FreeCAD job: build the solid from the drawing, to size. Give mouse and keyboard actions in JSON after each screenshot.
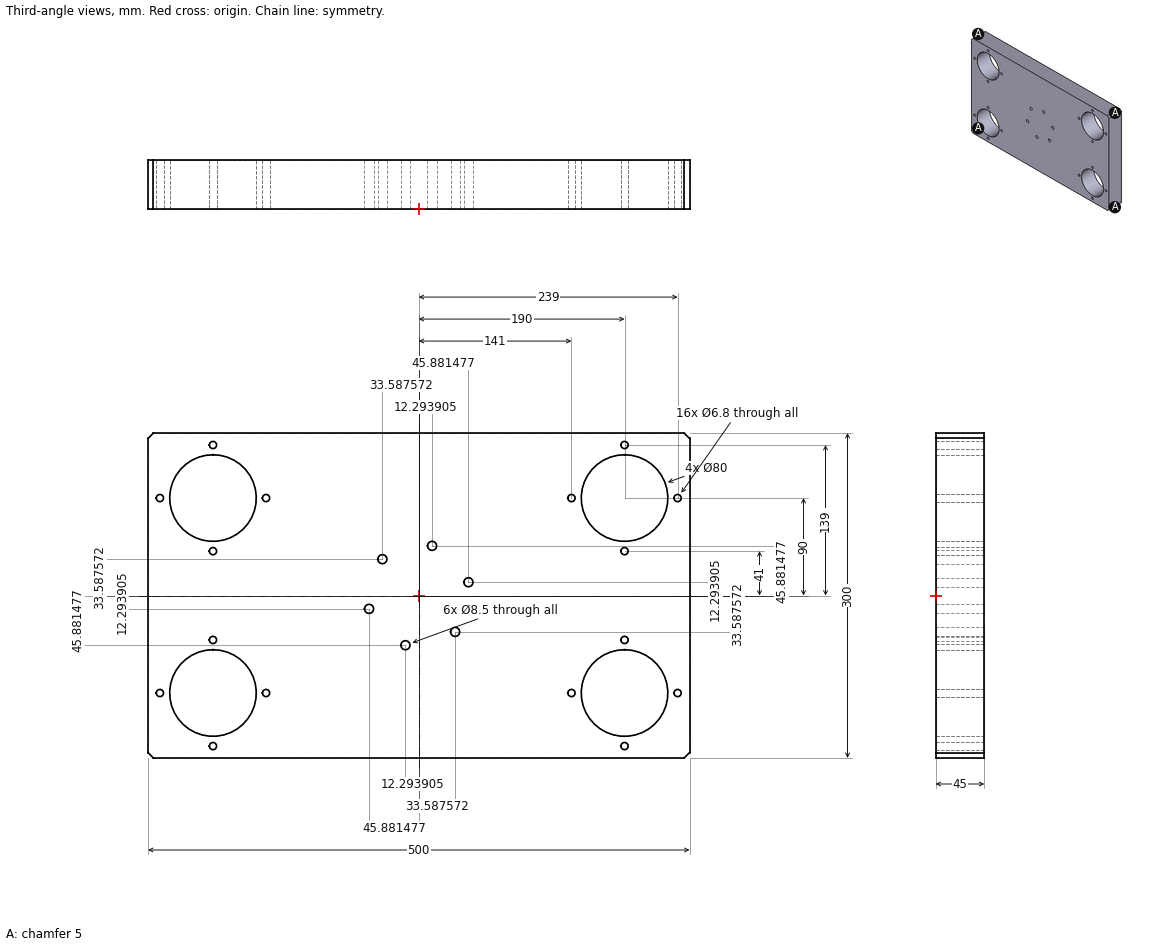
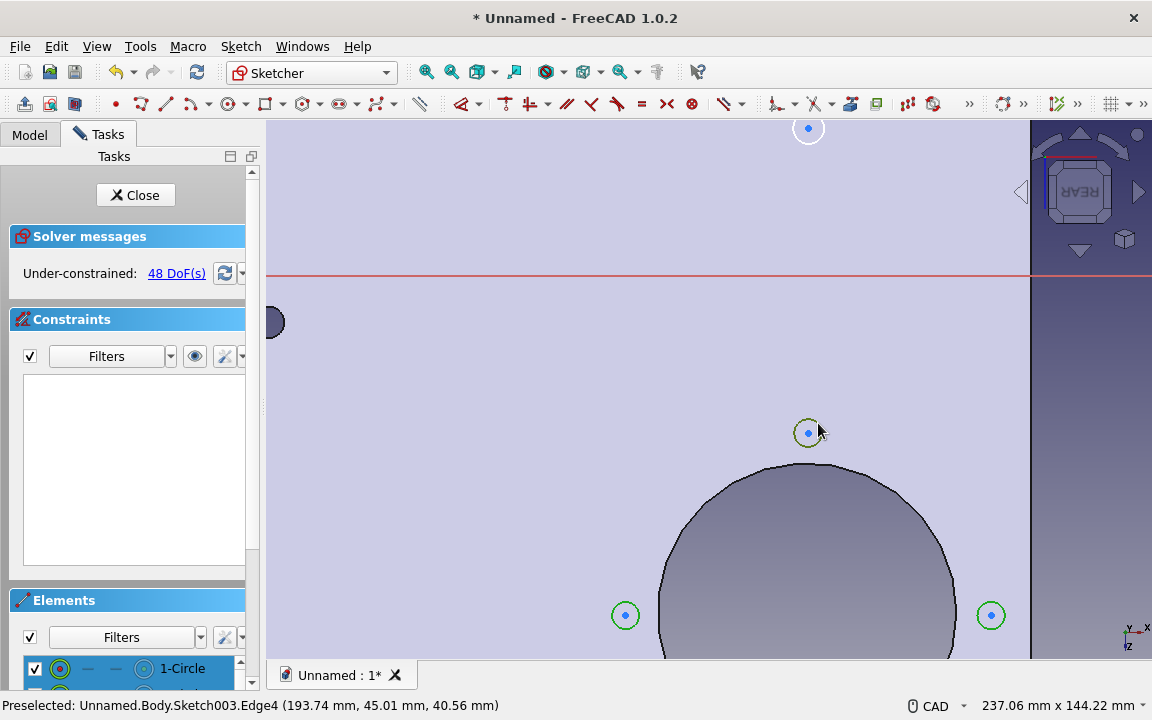
{"action": "scroll", "coordinate": [818, 427], "scroll_direction": "down", "scroll_amount": 7}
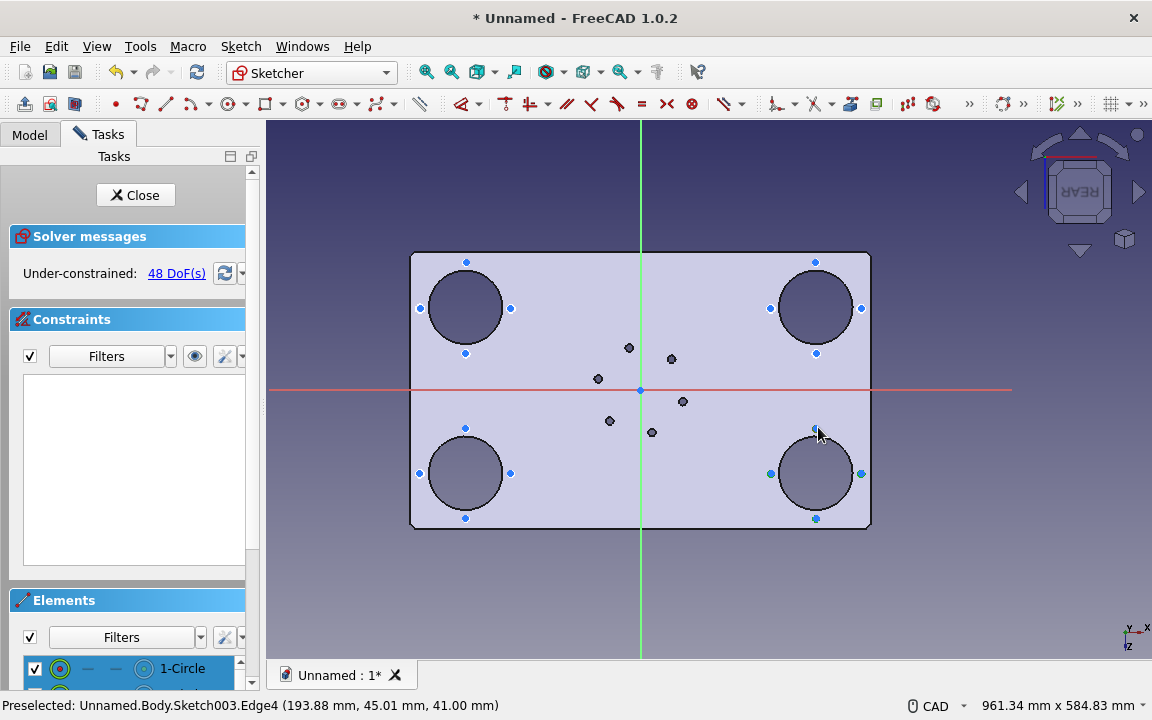
{"action": "scroll", "coordinate": [864, 306], "scroll_direction": "up", "scroll_amount": 7}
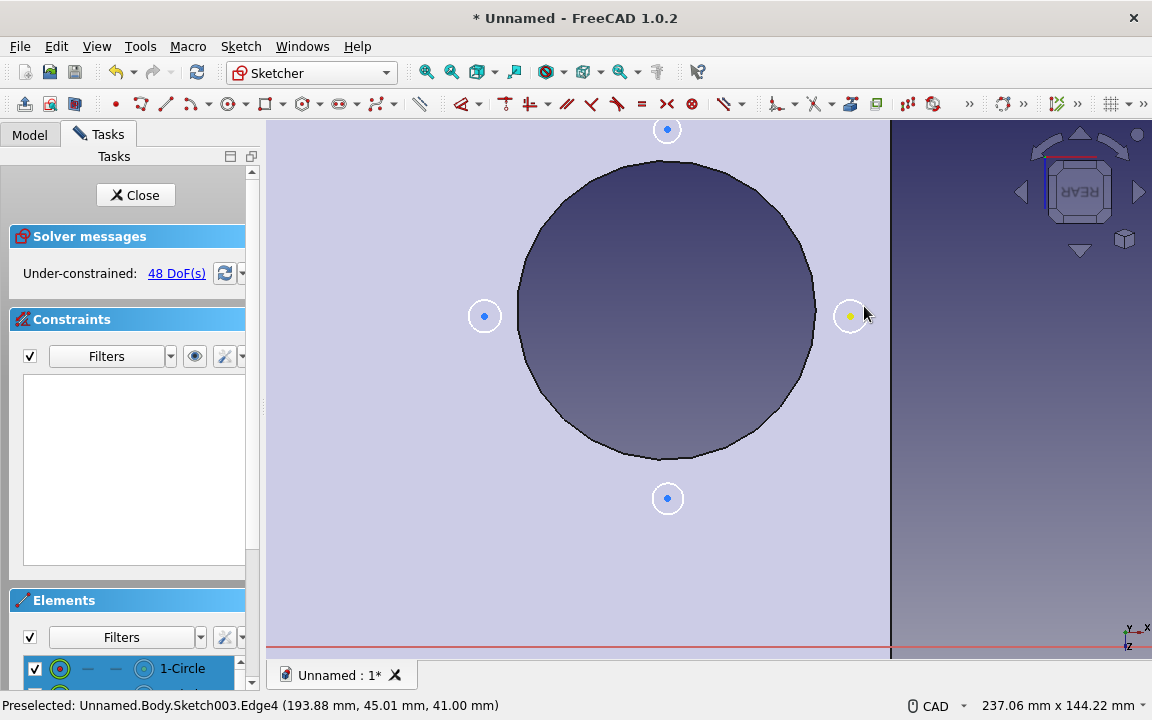
{"action": "left_click", "coordinate": [862, 305]}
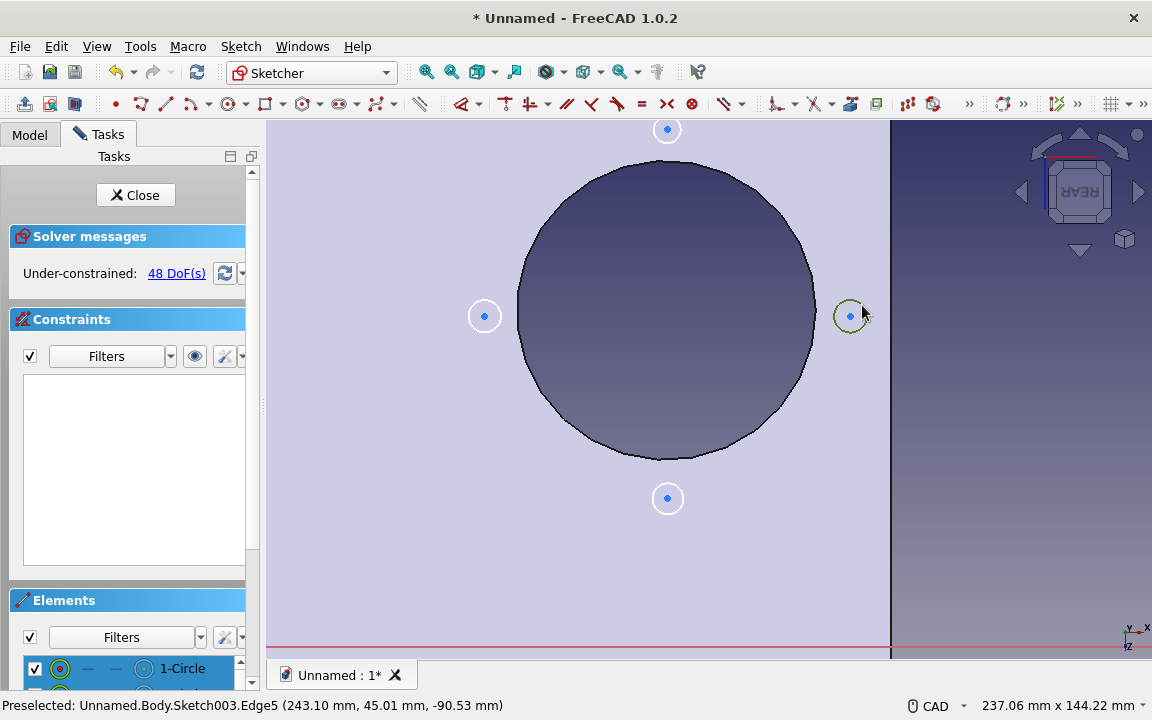
{"action": "left_click", "coordinate": [679, 488]}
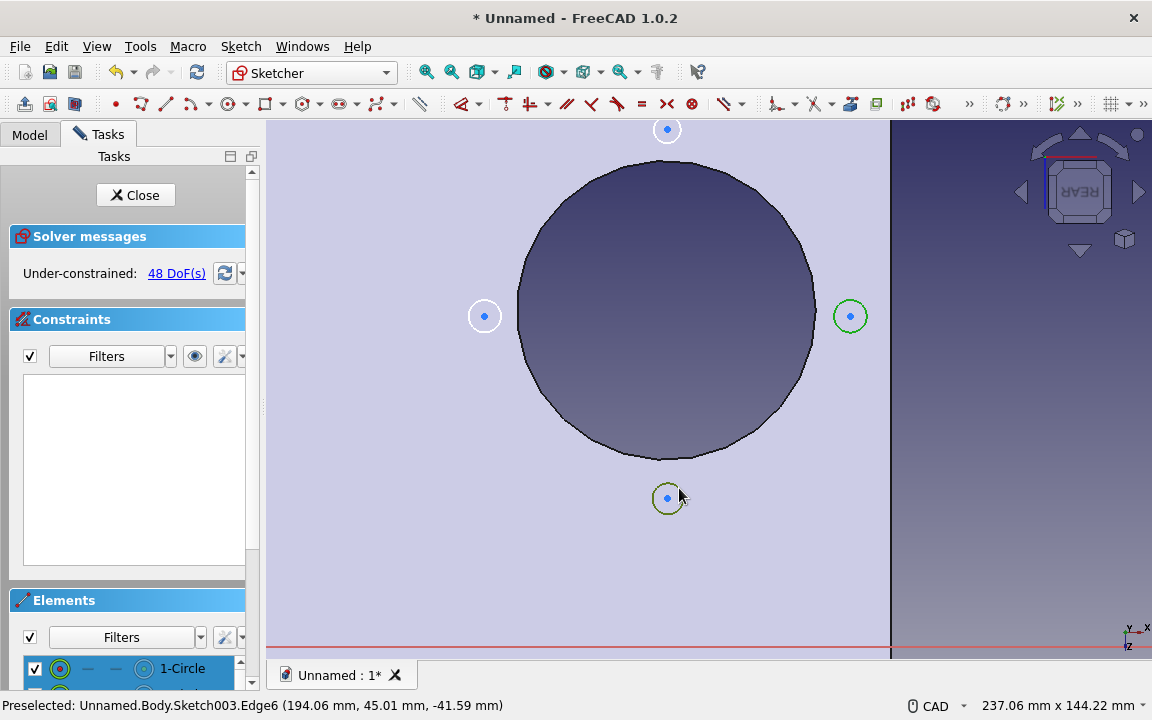
{"action": "left_click", "coordinate": [496, 305]}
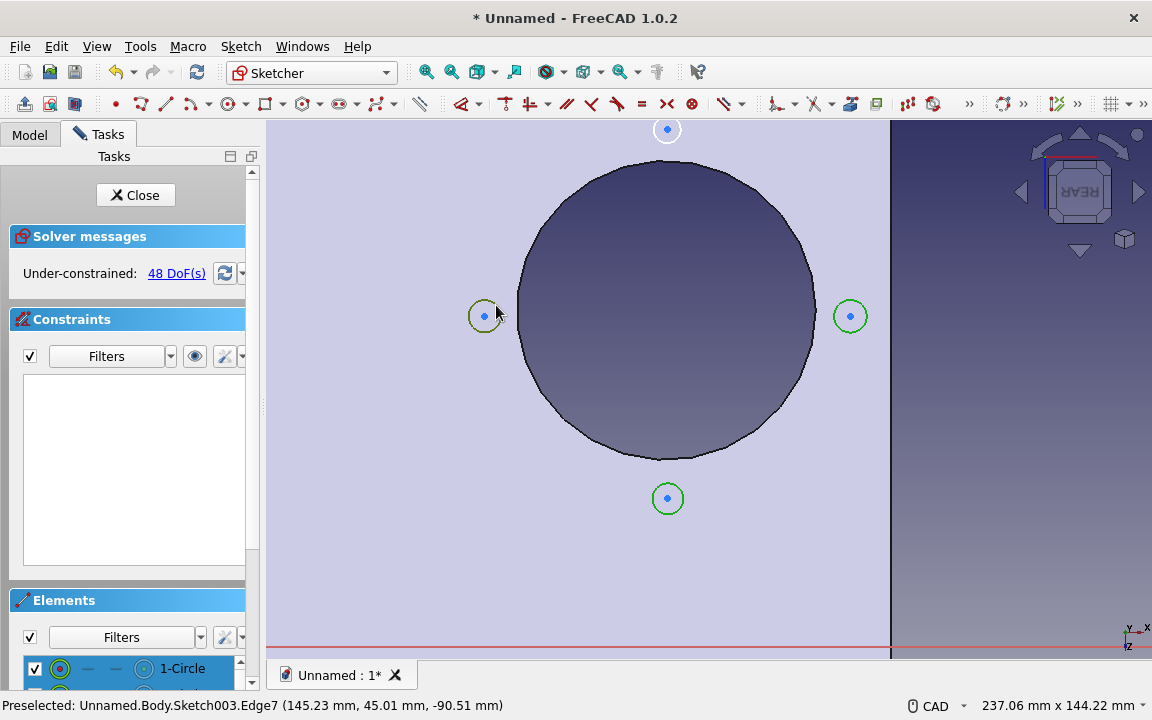
{"action": "scroll", "coordinate": [864, 305], "scroll_direction": "down", "scroll_amount": 7}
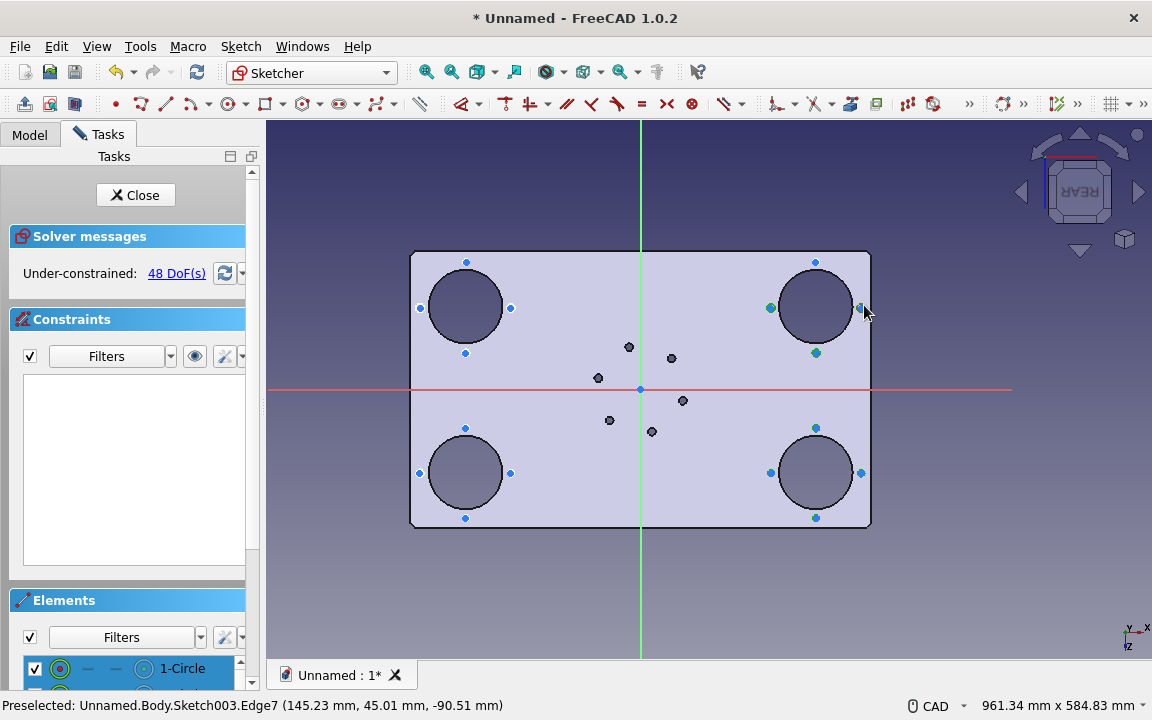
{"action": "scroll", "coordinate": [818, 260], "scroll_direction": "up", "scroll_amount": 8}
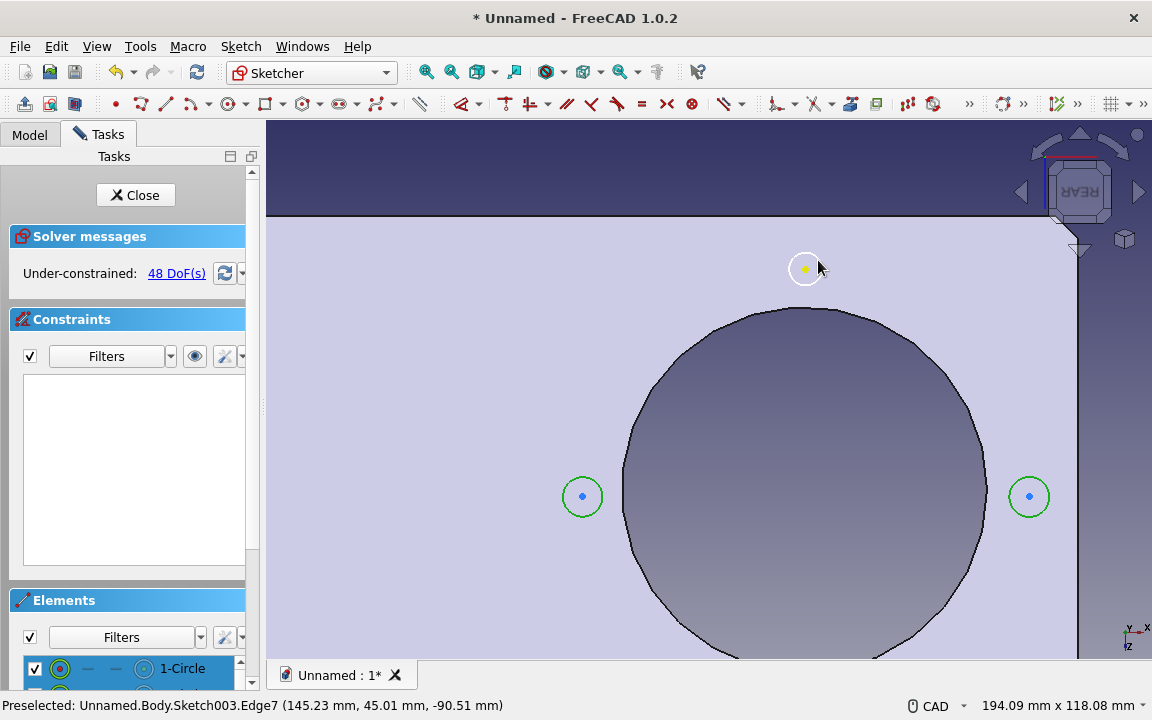
{"action": "left_click", "coordinate": [817, 257]}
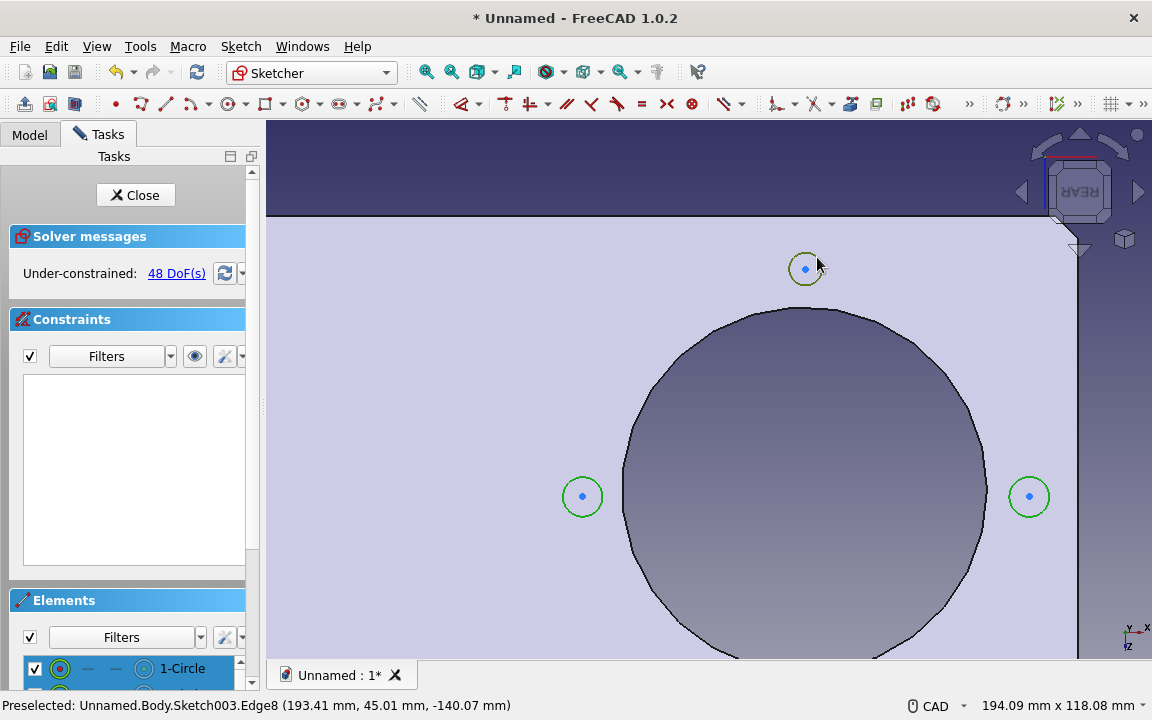
{"action": "scroll", "coordinate": [818, 260], "scroll_direction": "down", "scroll_amount": 8}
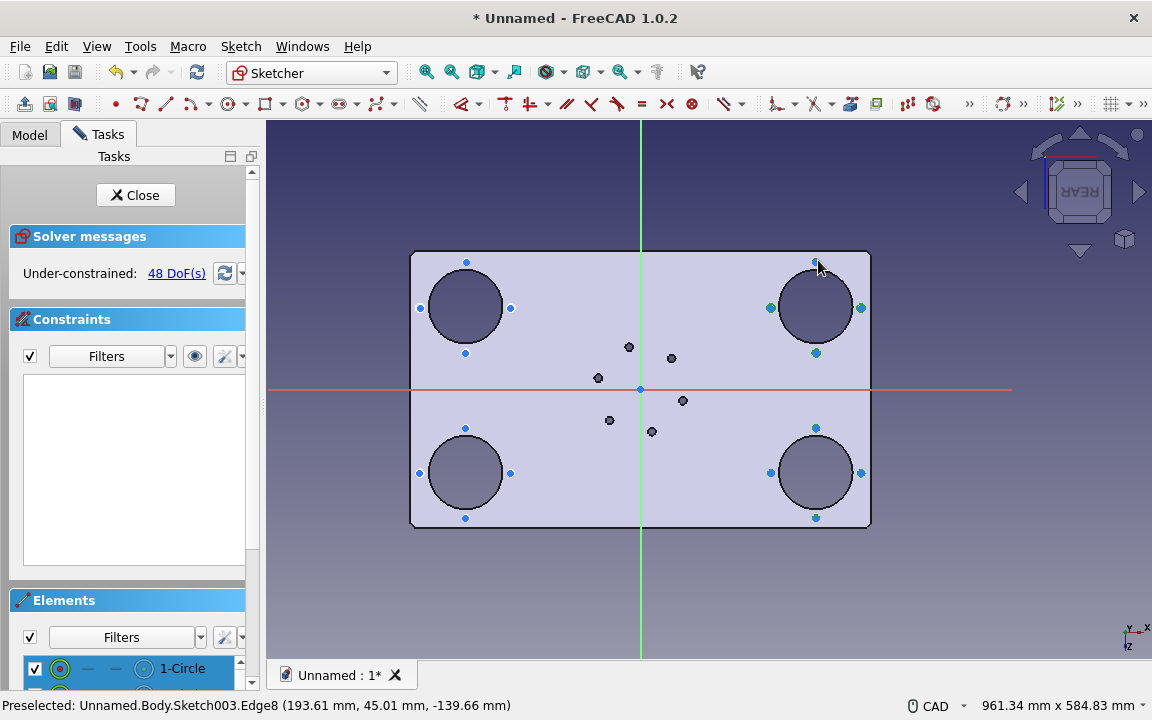
{"action": "scroll", "coordinate": [513, 471], "scroll_direction": "up", "scroll_amount": 8}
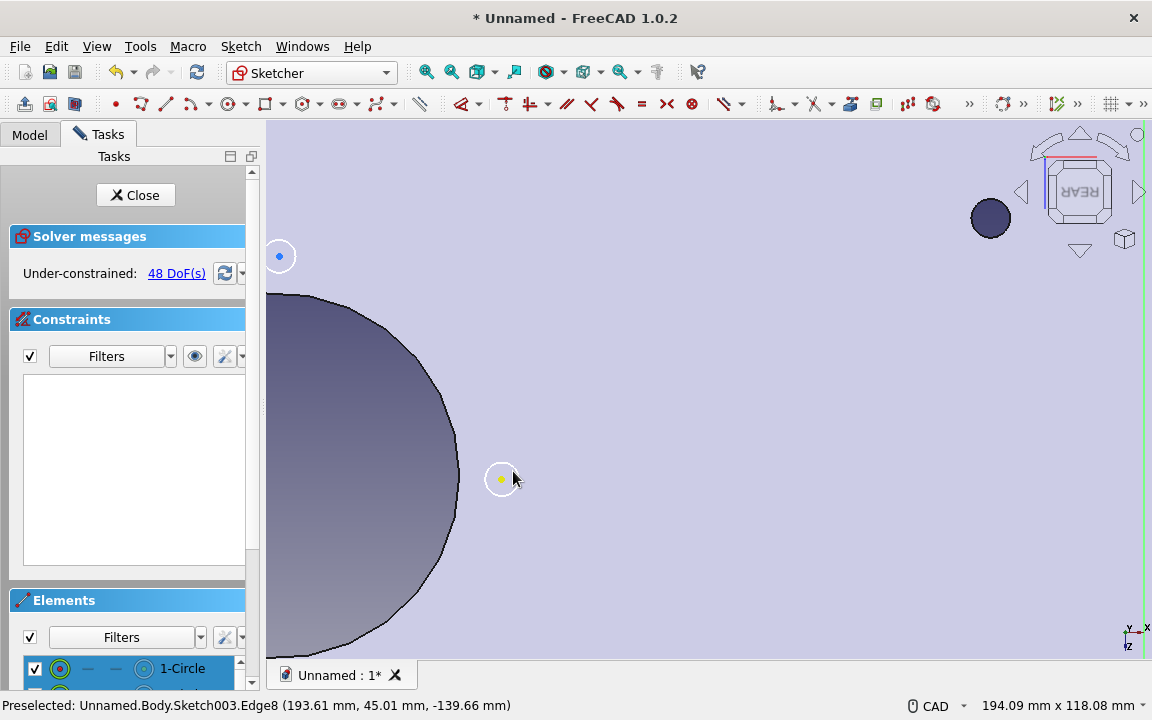
{"action": "left_click", "coordinate": [514, 467]}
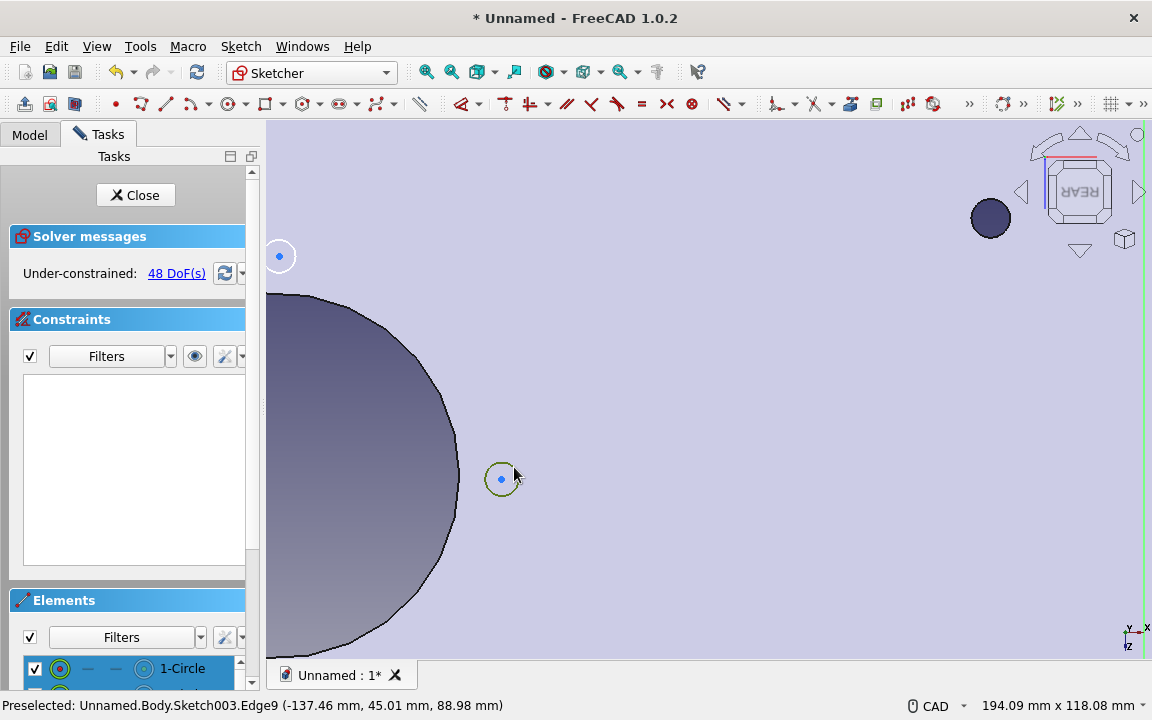
{"action": "scroll", "coordinate": [513, 472], "scroll_direction": "down", "scroll_amount": 8}